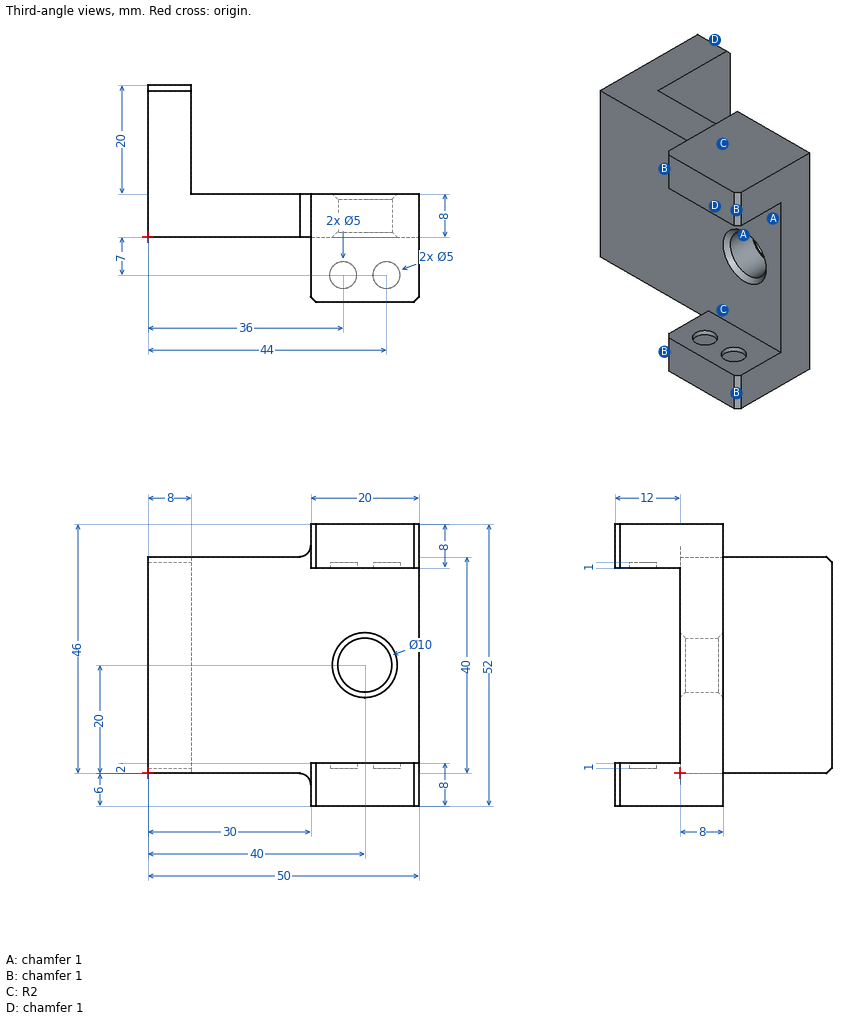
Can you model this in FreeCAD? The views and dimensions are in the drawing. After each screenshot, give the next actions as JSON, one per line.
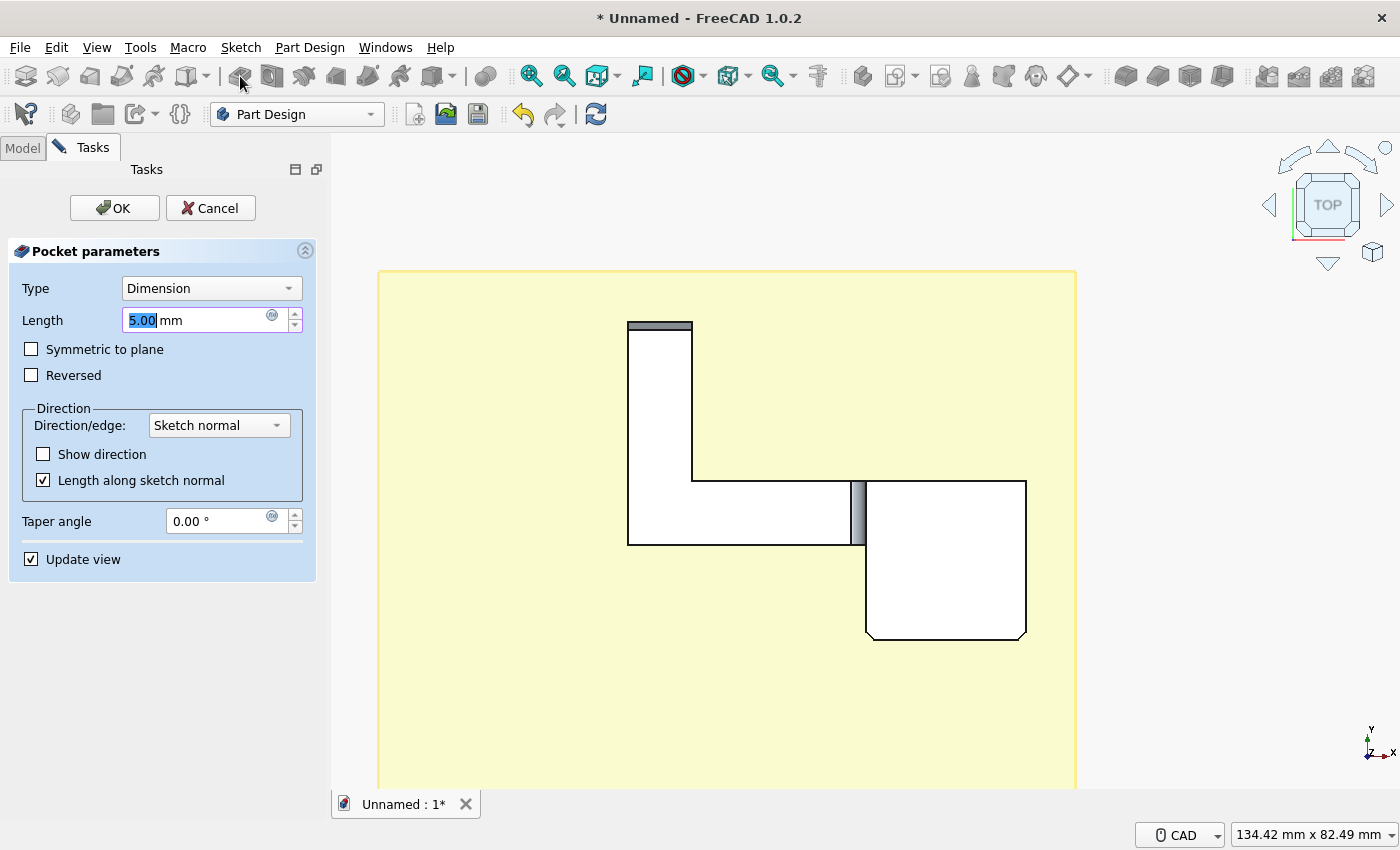
{"action": "type", "text": "1"}
{"action": "key", "text": "Tab"}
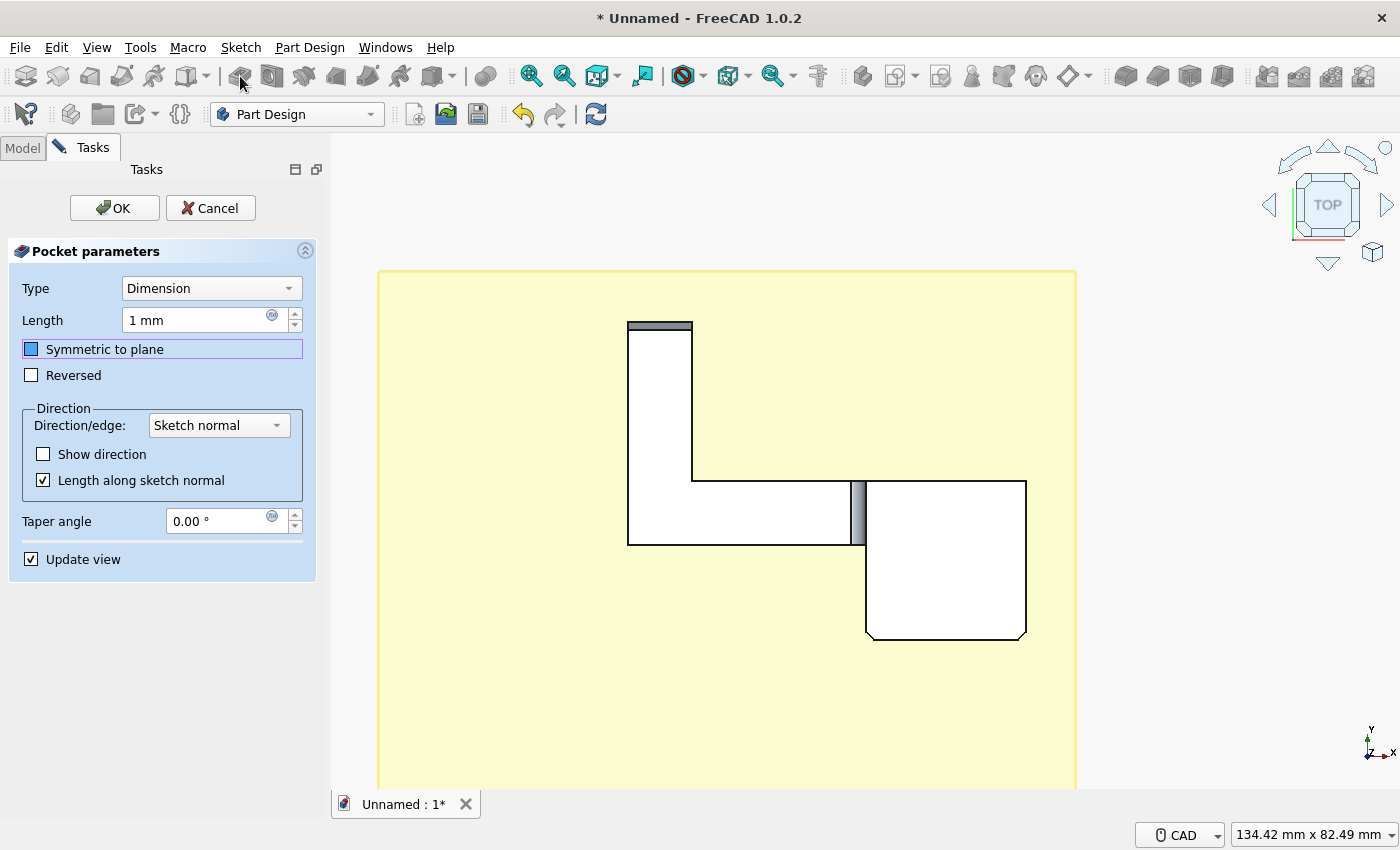
{"action": "left_click", "coordinate": [115, 208]}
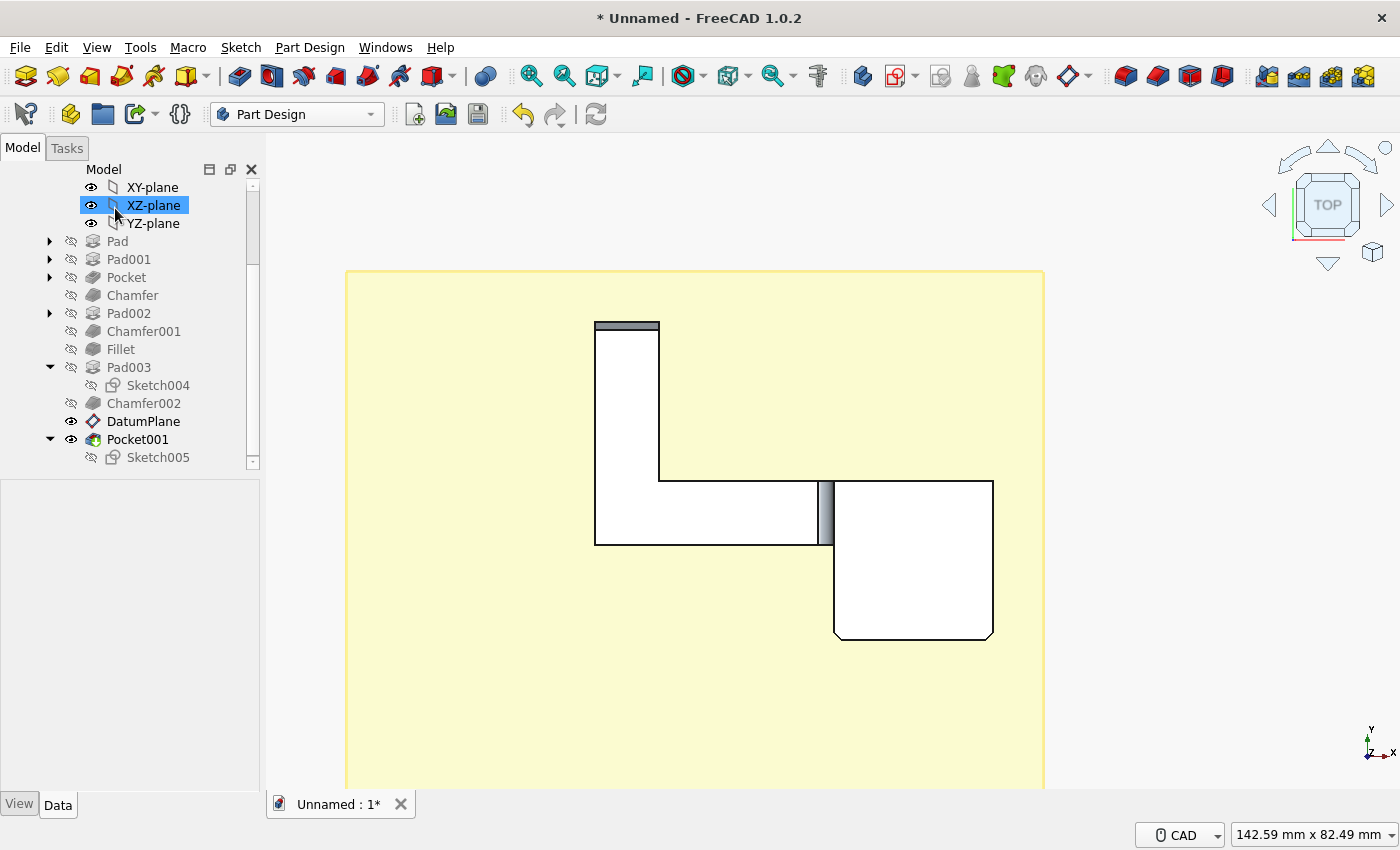
{"action": "left_click", "coordinate": [116, 421]}
{"action": "key", "text": "space"}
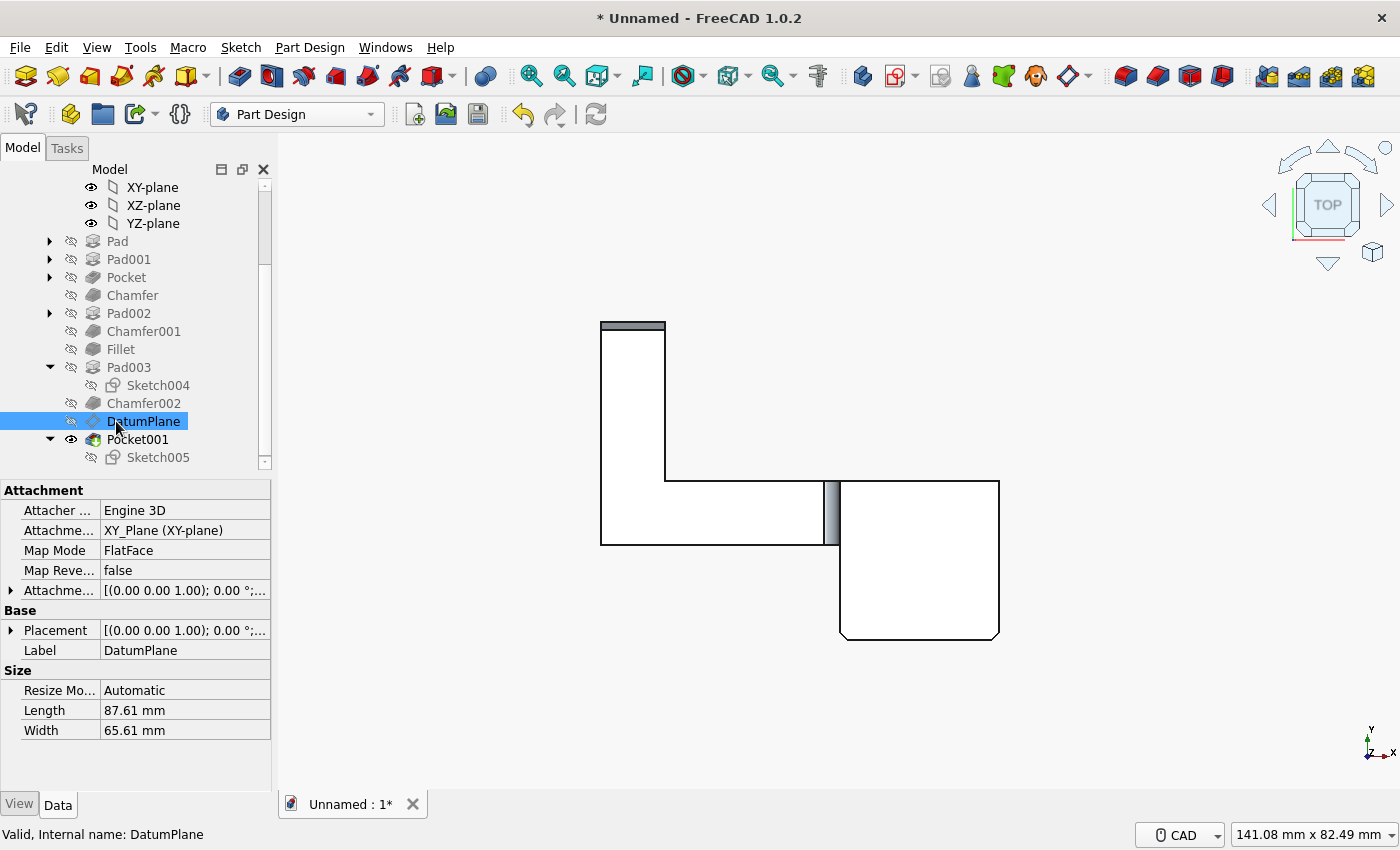
{"action": "scroll", "coordinate": [160, 327], "scroll_direction": "down", "scroll_amount": 3}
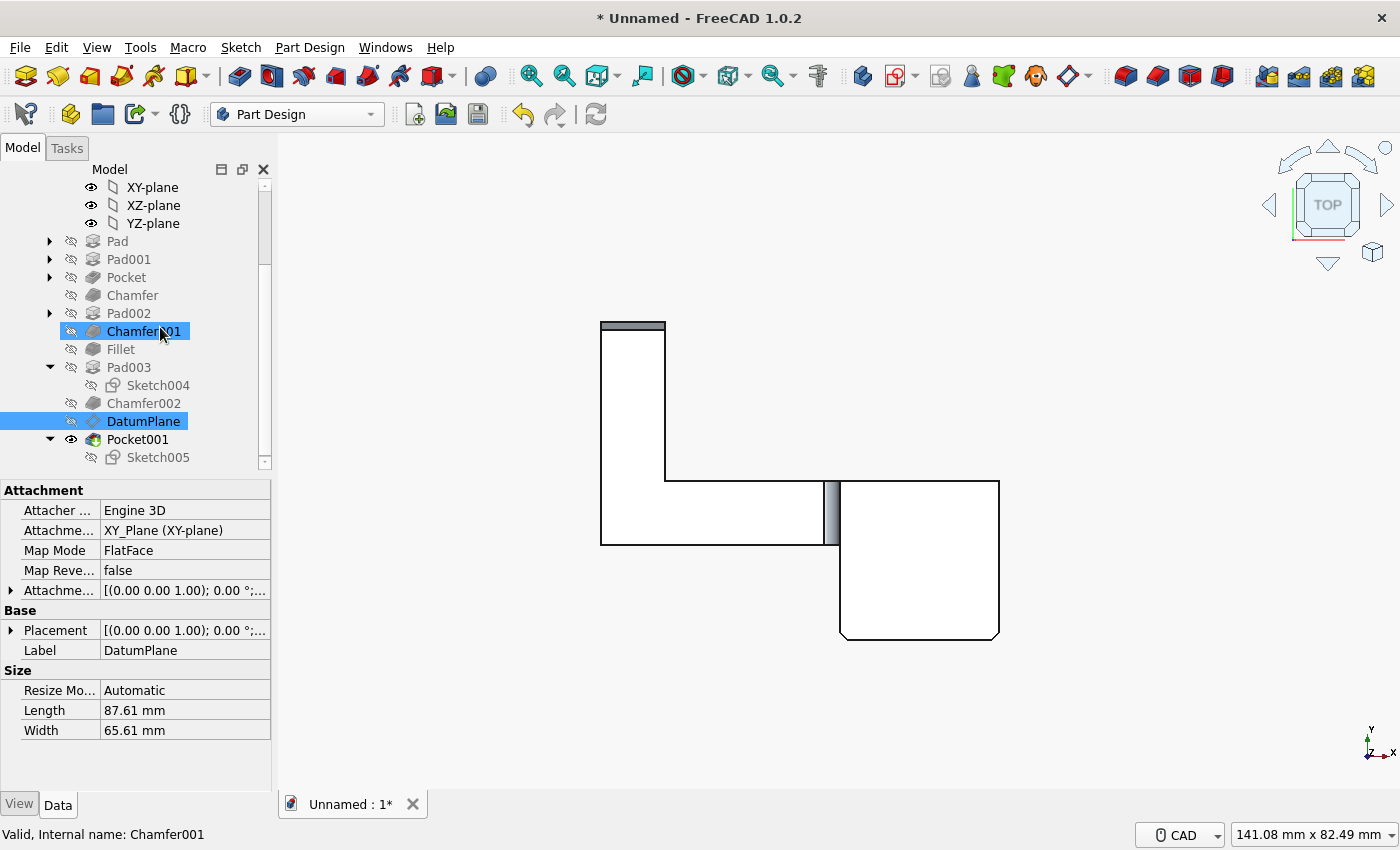
{"action": "scroll", "coordinate": [160, 327], "scroll_direction": "up", "scroll_amount": 15}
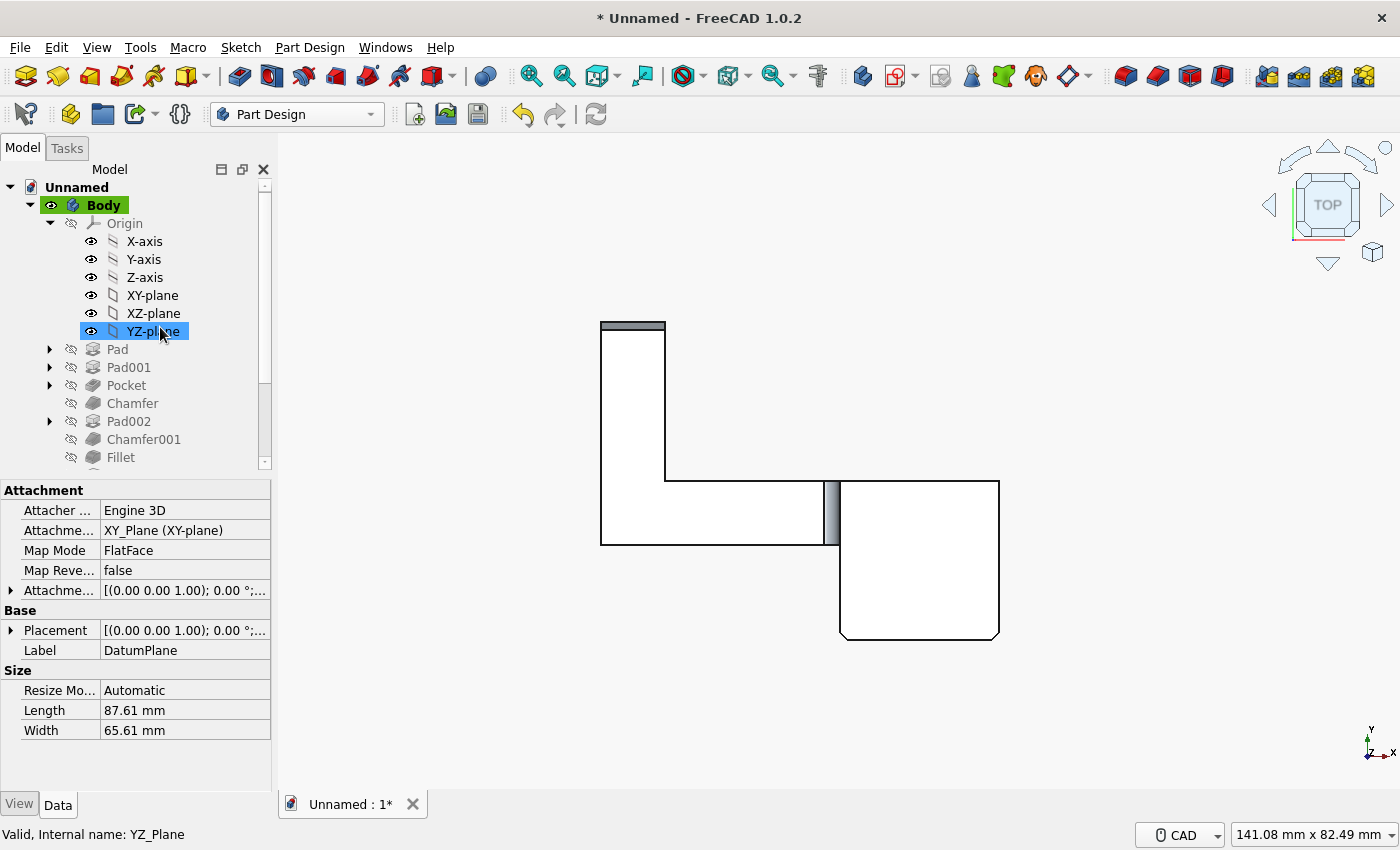
{"action": "left_click", "coordinate": [136, 295]}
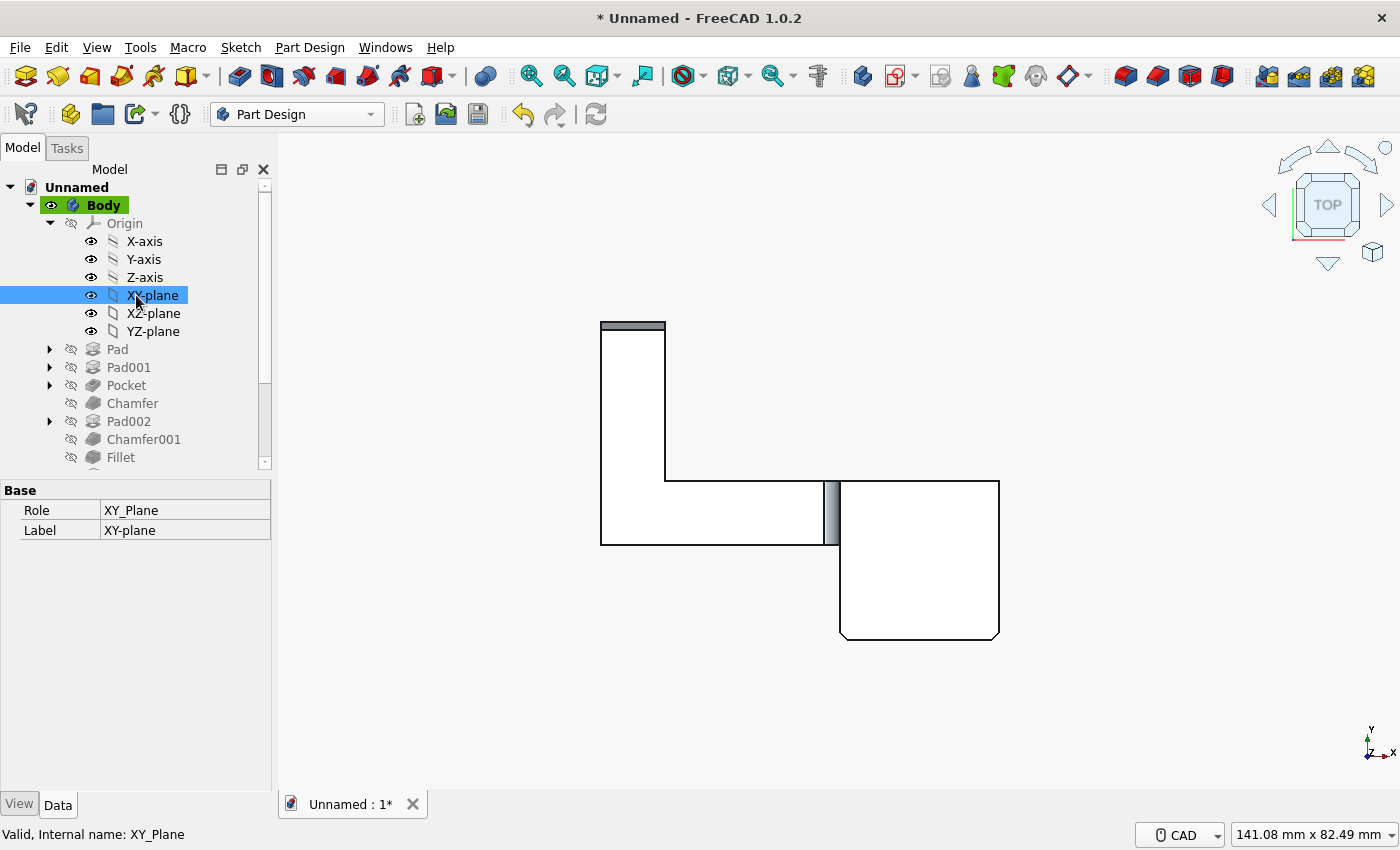
{"action": "left_click", "coordinate": [1068, 76]}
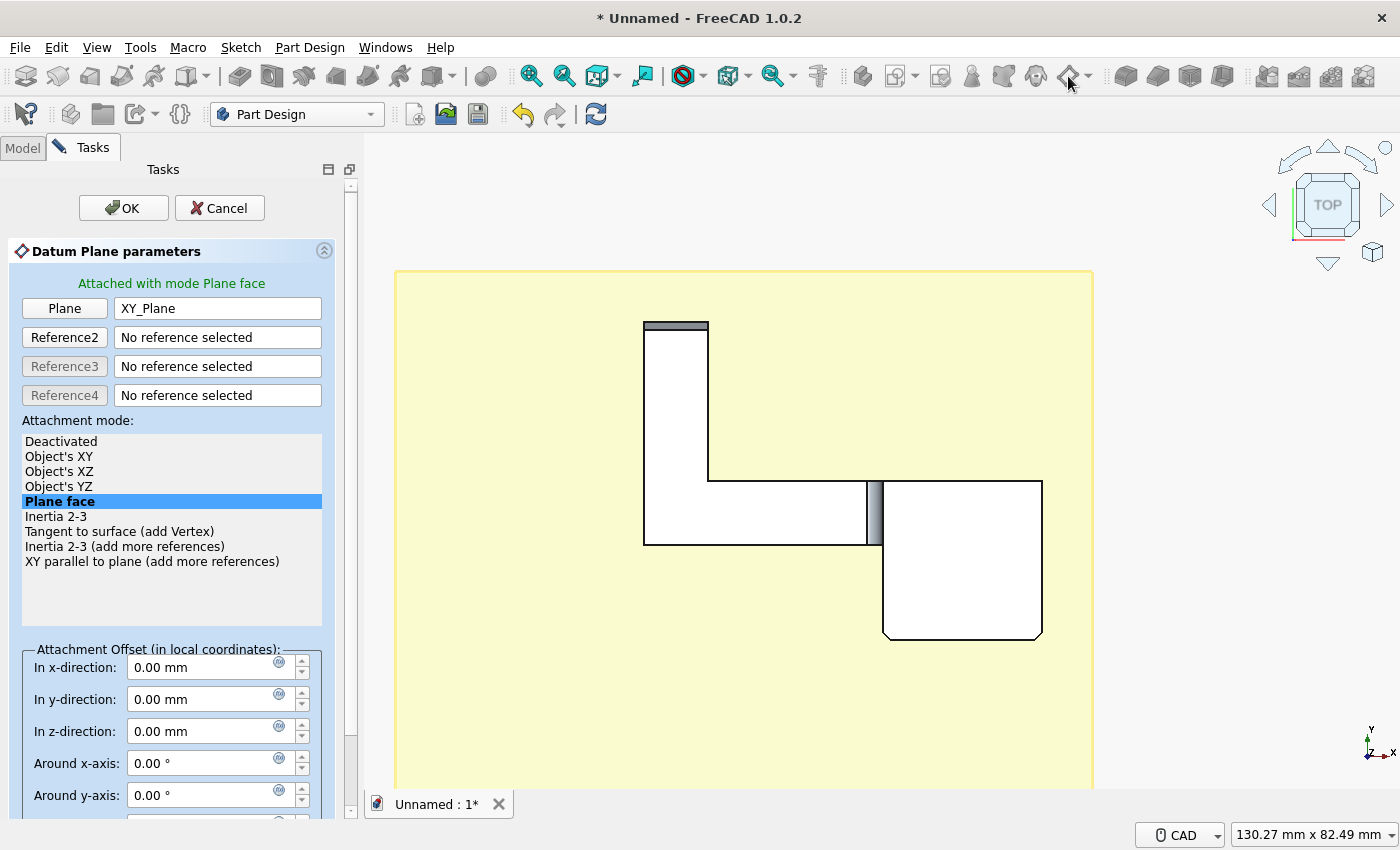
{"action": "triple_click", "coordinate": [210, 731]}